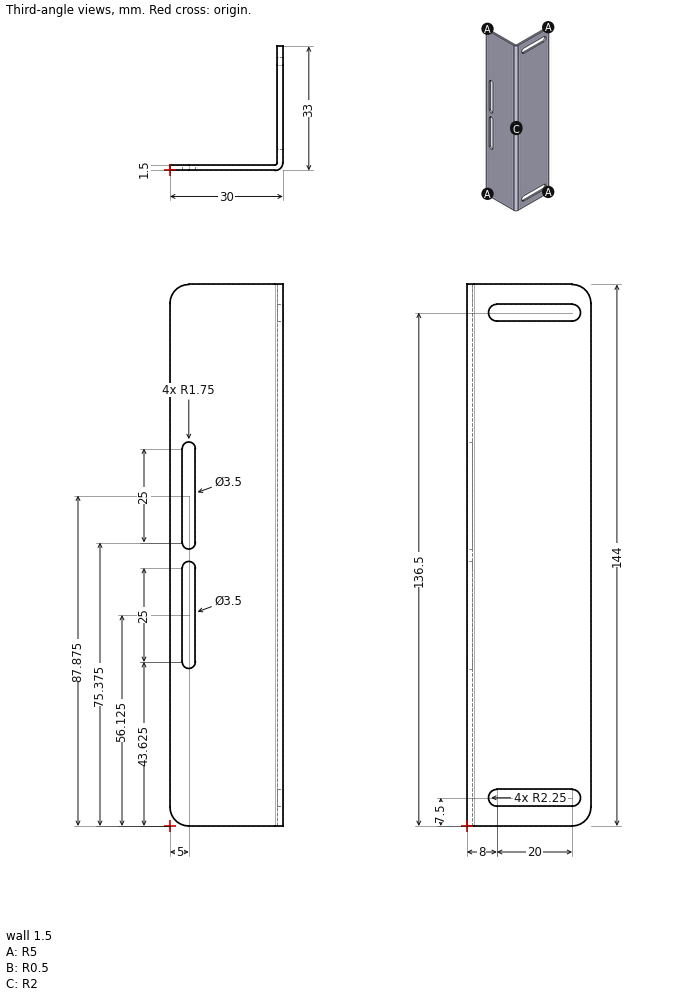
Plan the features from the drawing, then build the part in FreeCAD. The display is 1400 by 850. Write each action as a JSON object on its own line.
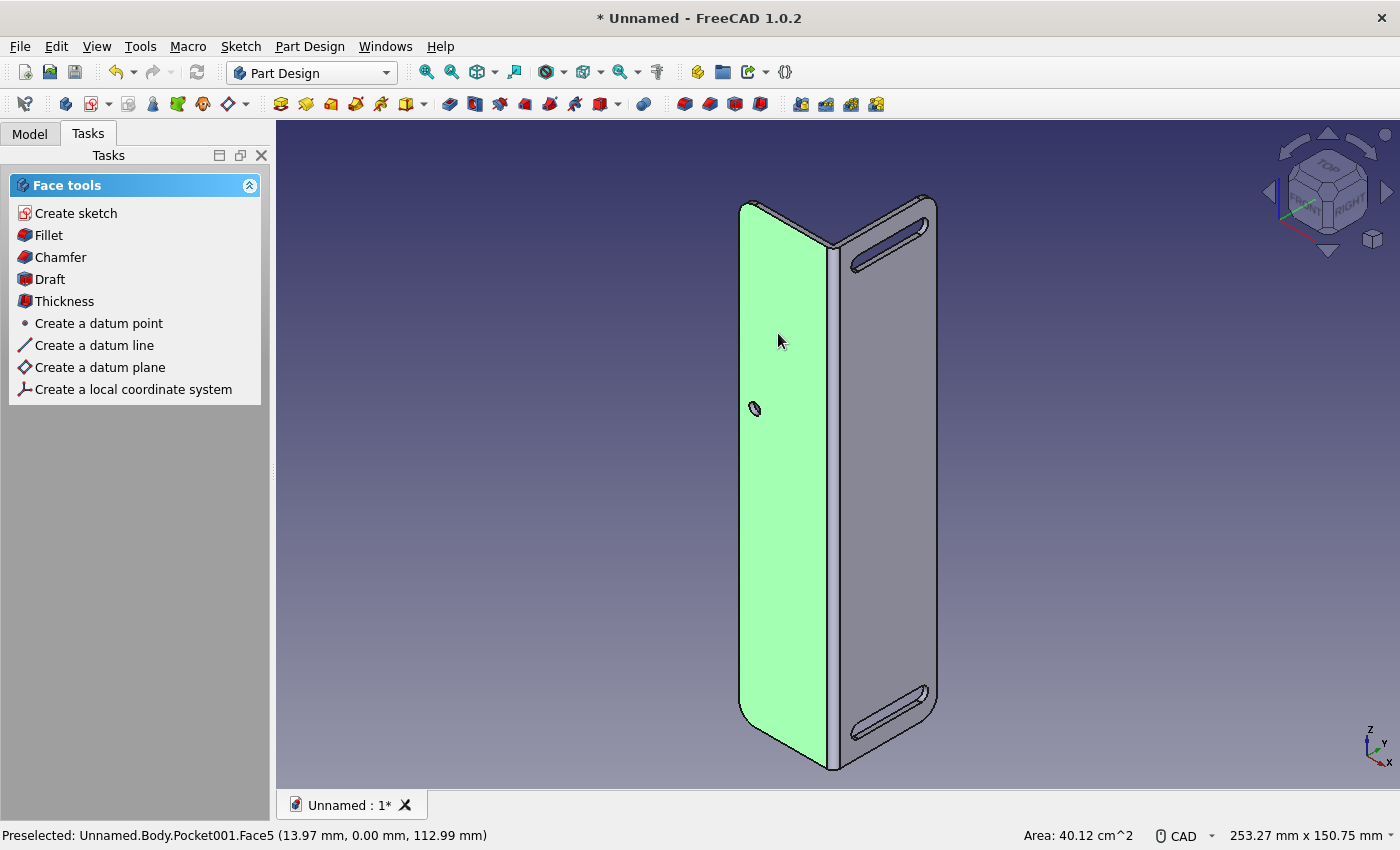
{"action": "left_click", "coordinate": [90, 104]}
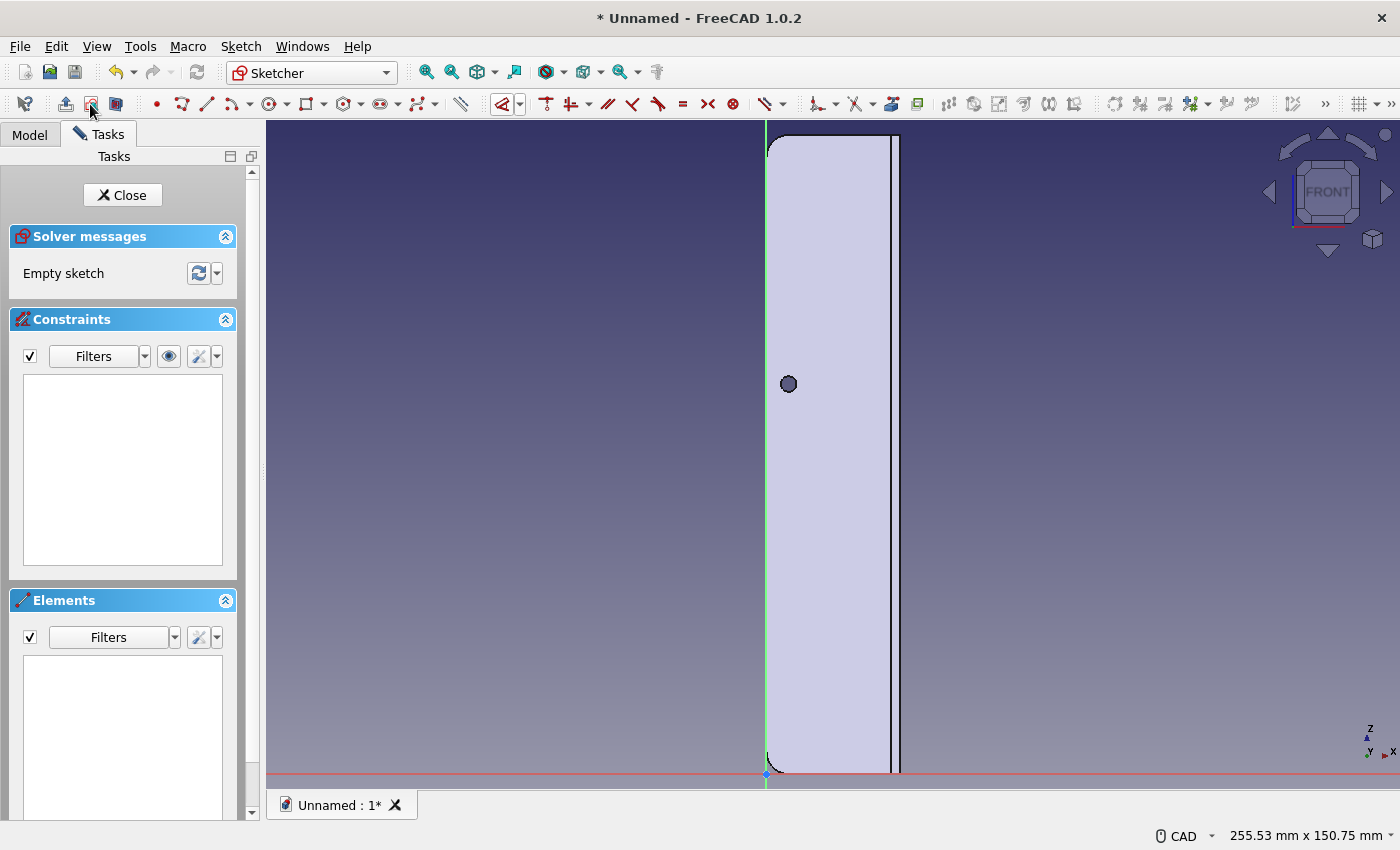
{"action": "scroll", "coordinate": [790, 529], "scroll_direction": "up", "scroll_amount": 15}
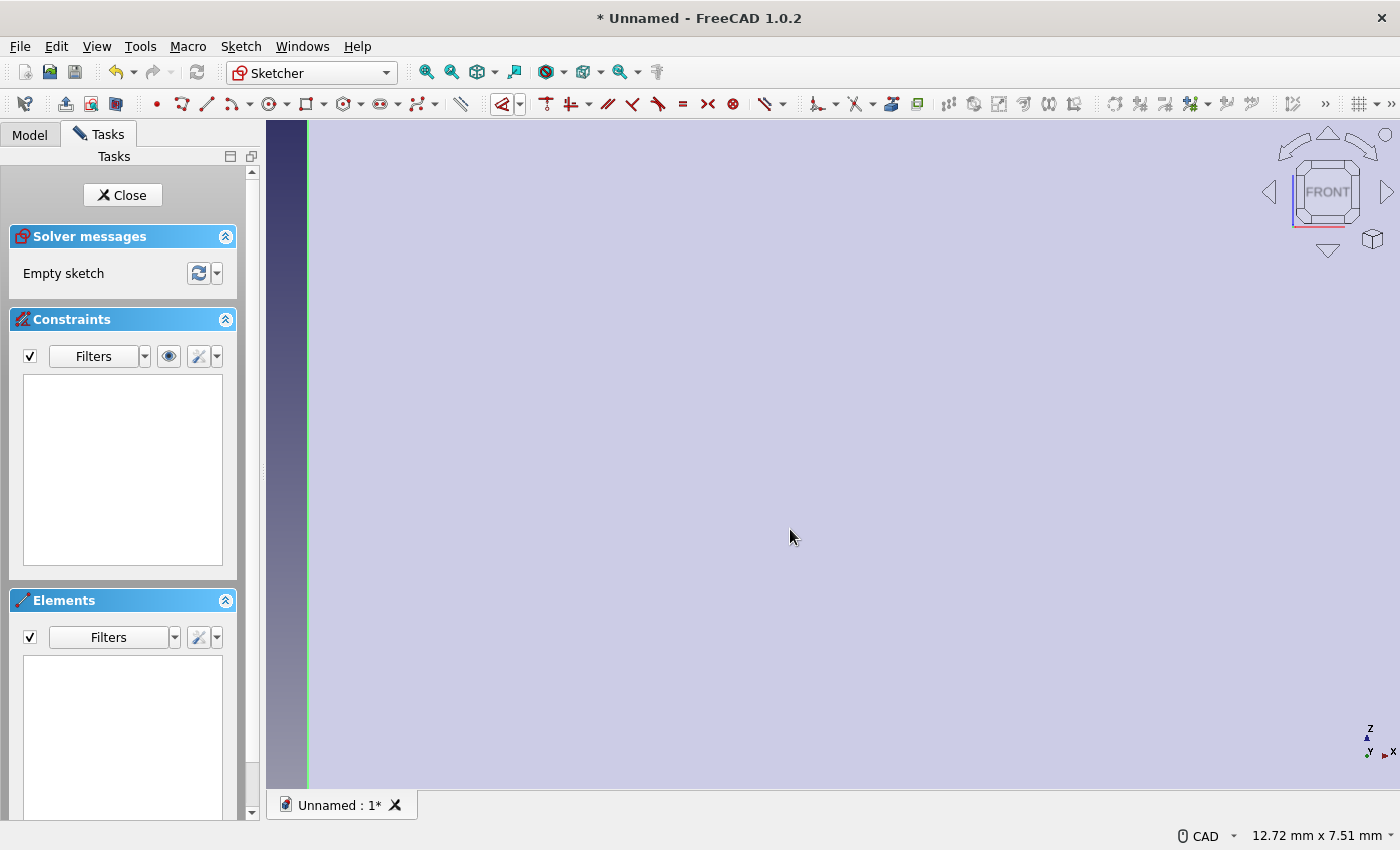
{"action": "scroll", "coordinate": [731, 398], "scroll_direction": "up", "scroll_amount": 2}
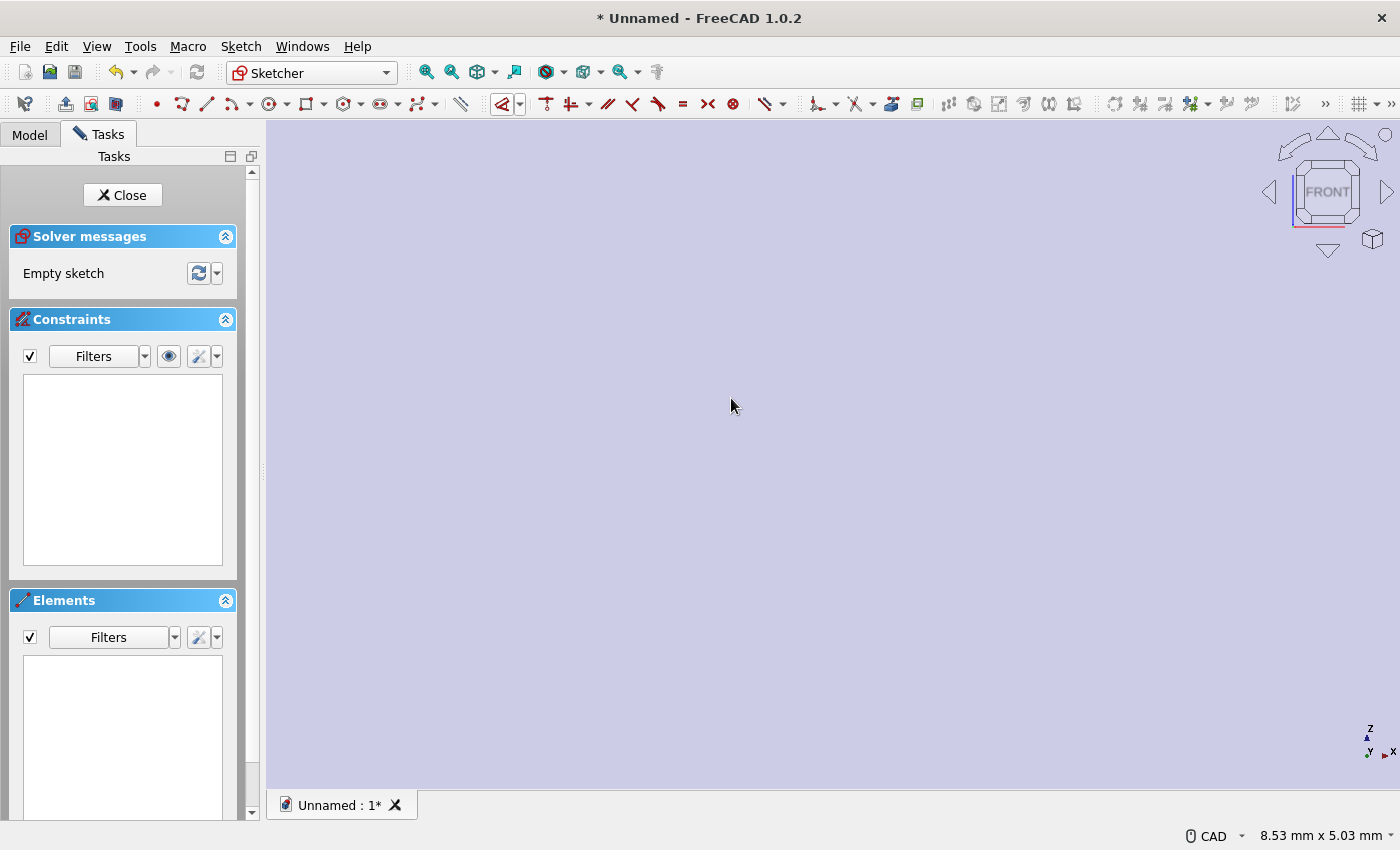
{"action": "left_click", "coordinate": [268, 104]}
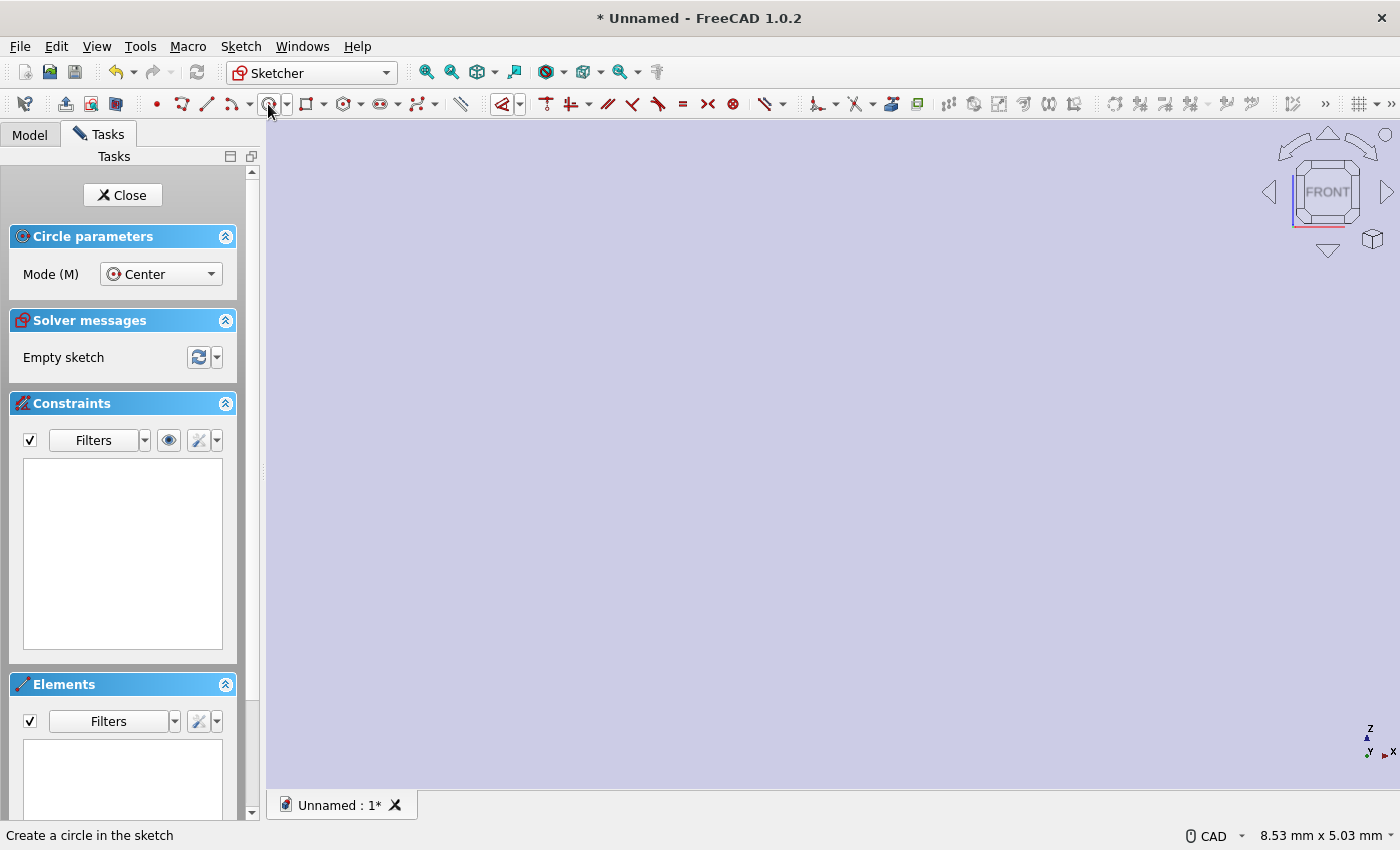
{"action": "left_click", "coordinate": [764, 454]}
{"action": "left_click", "coordinate": [929, 290]}
{"action": "key", "text": "Escape"}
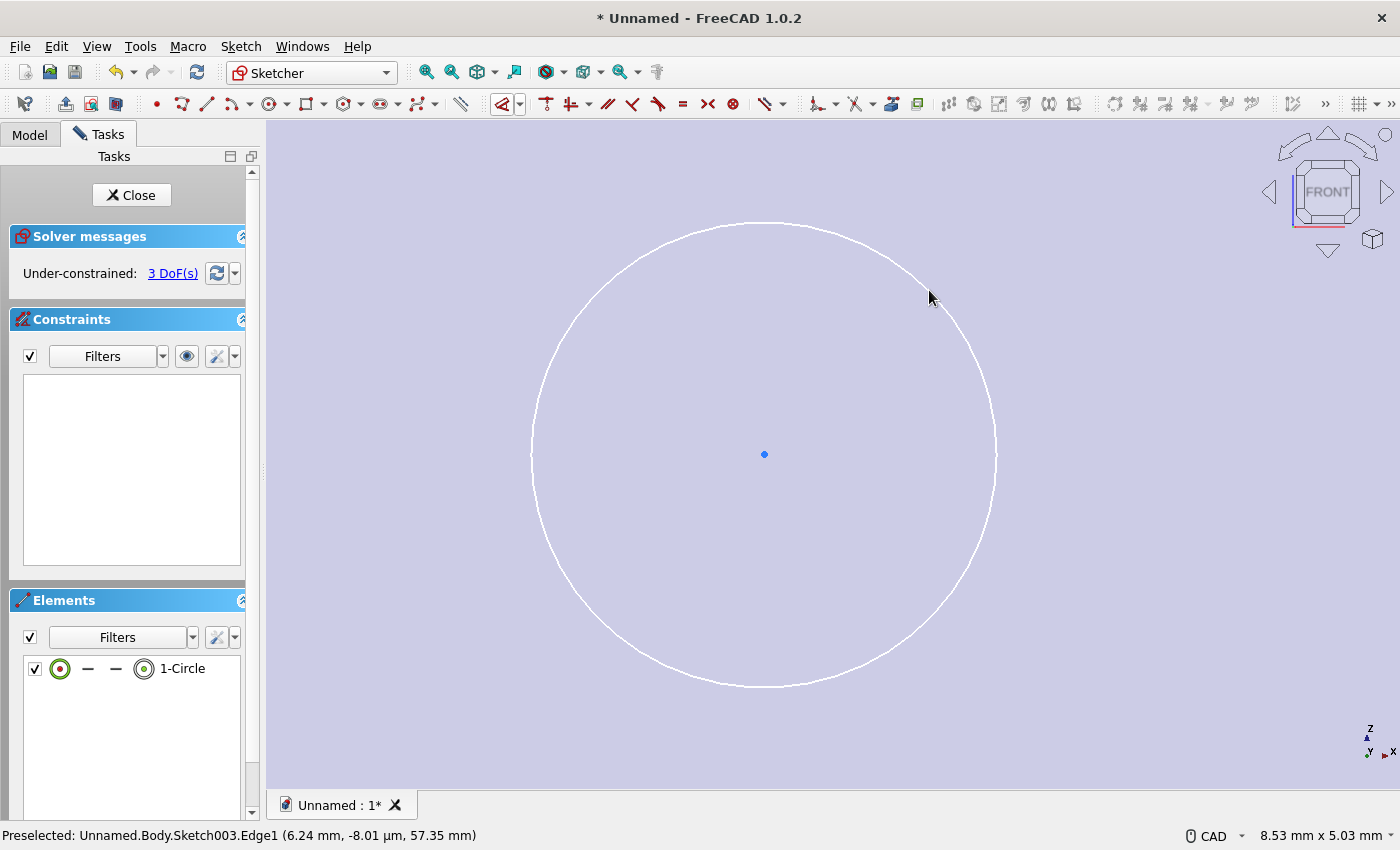
{"action": "left_click", "coordinate": [928, 290]}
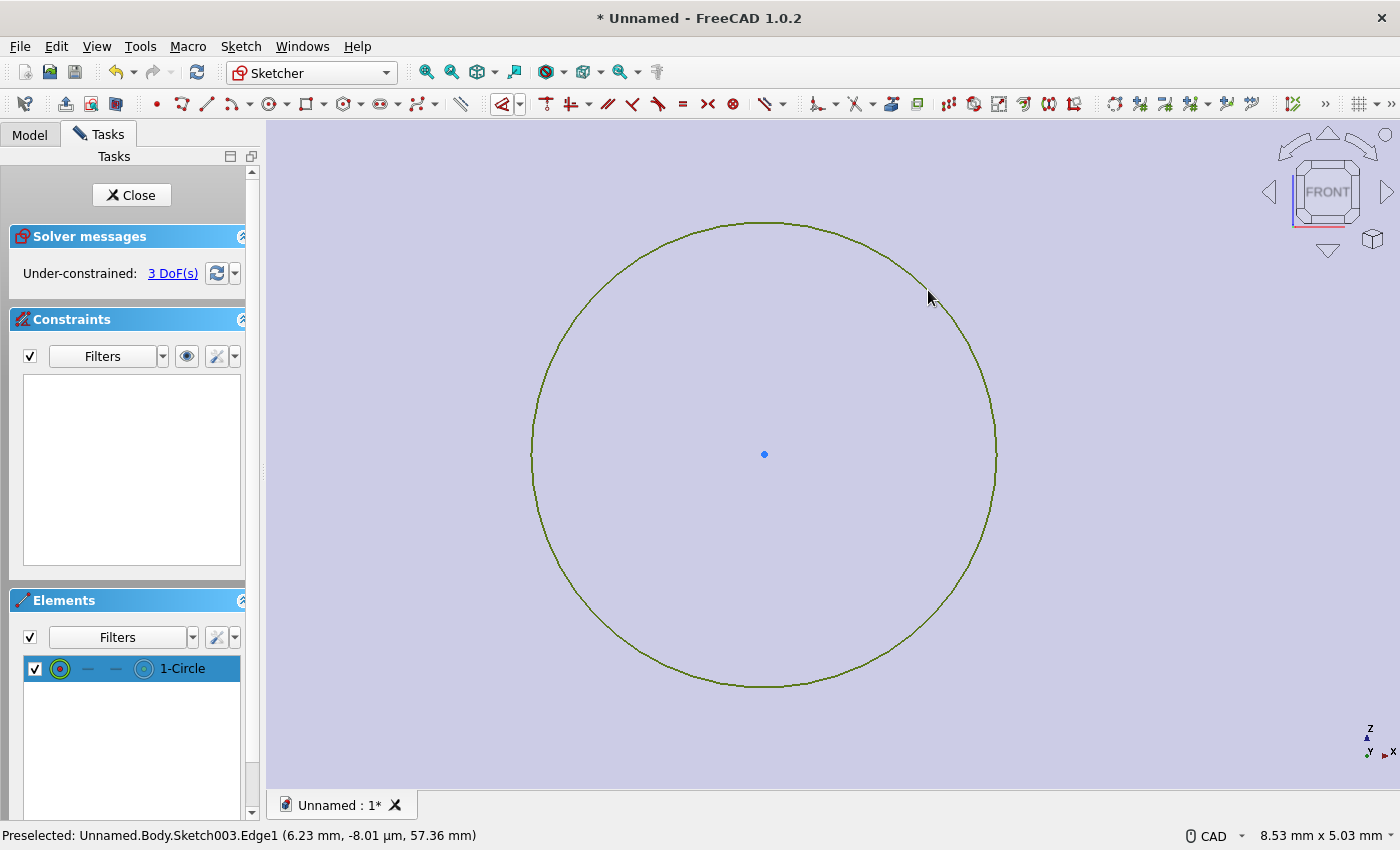
{"action": "left_click", "coordinate": [520, 104]}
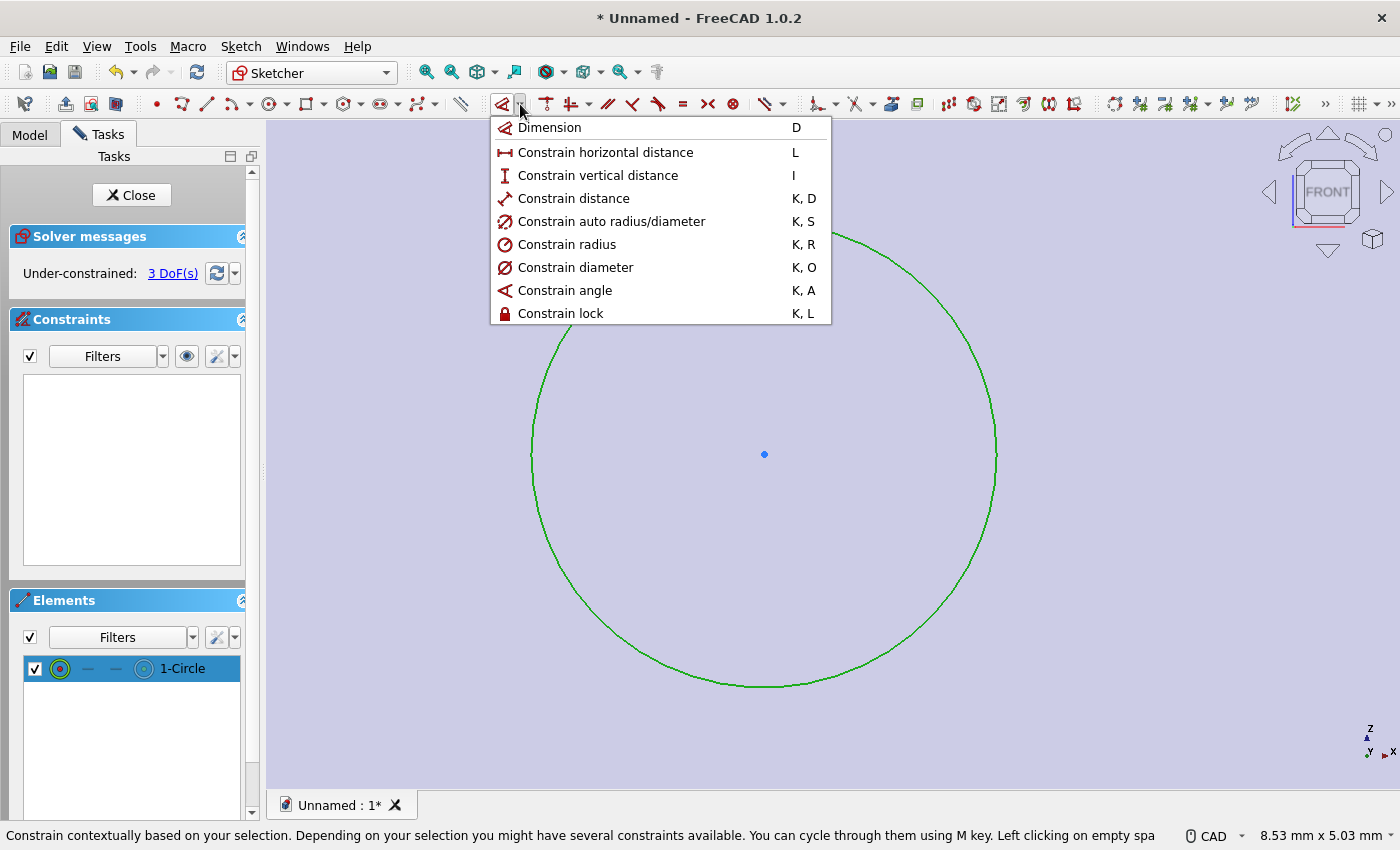
{"action": "left_click", "coordinate": [661, 268]}